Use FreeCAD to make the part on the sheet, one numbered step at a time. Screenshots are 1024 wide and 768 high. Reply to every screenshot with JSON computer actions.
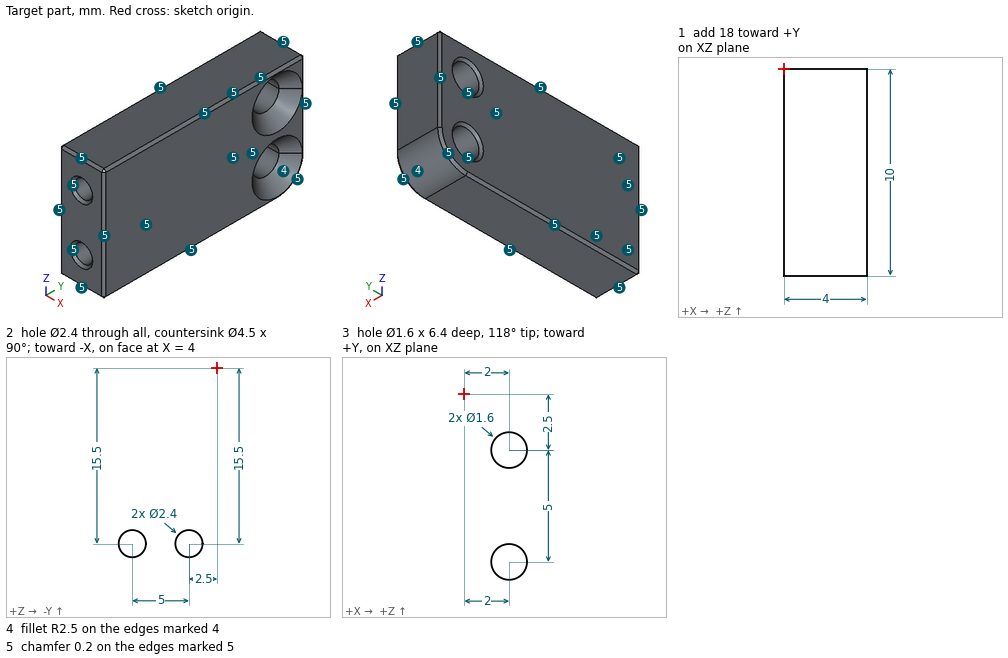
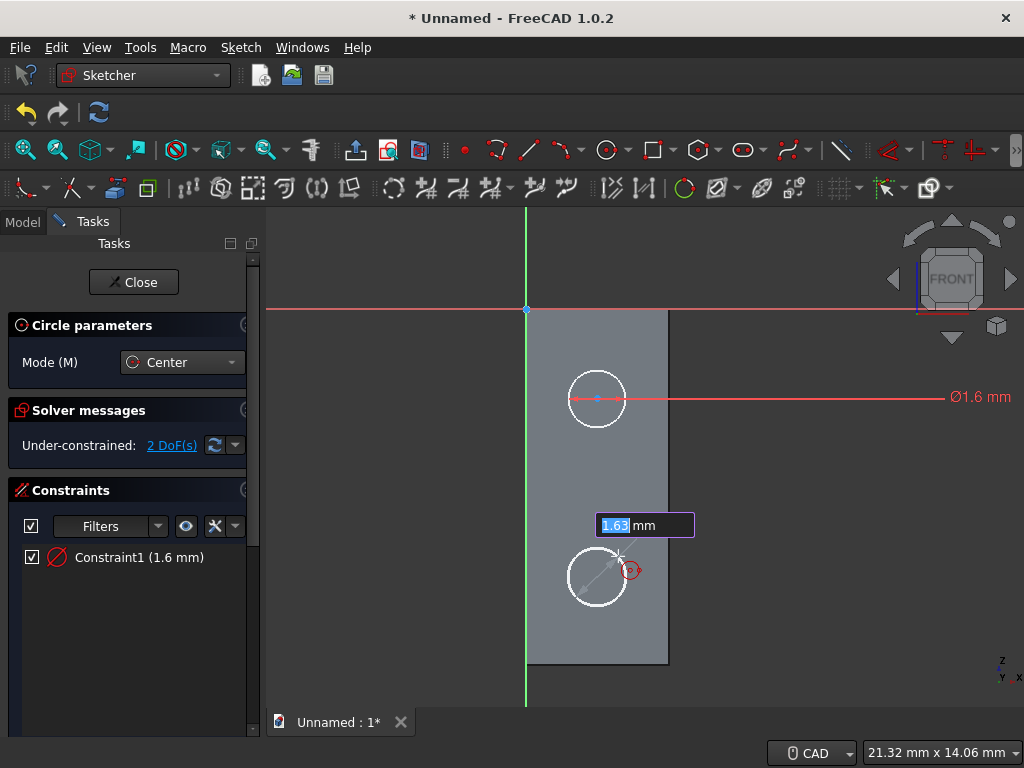
{"action": "type", "text": "1.6"}
{"action": "key", "text": "Return"}
{"action": "key", "text": "Escape"}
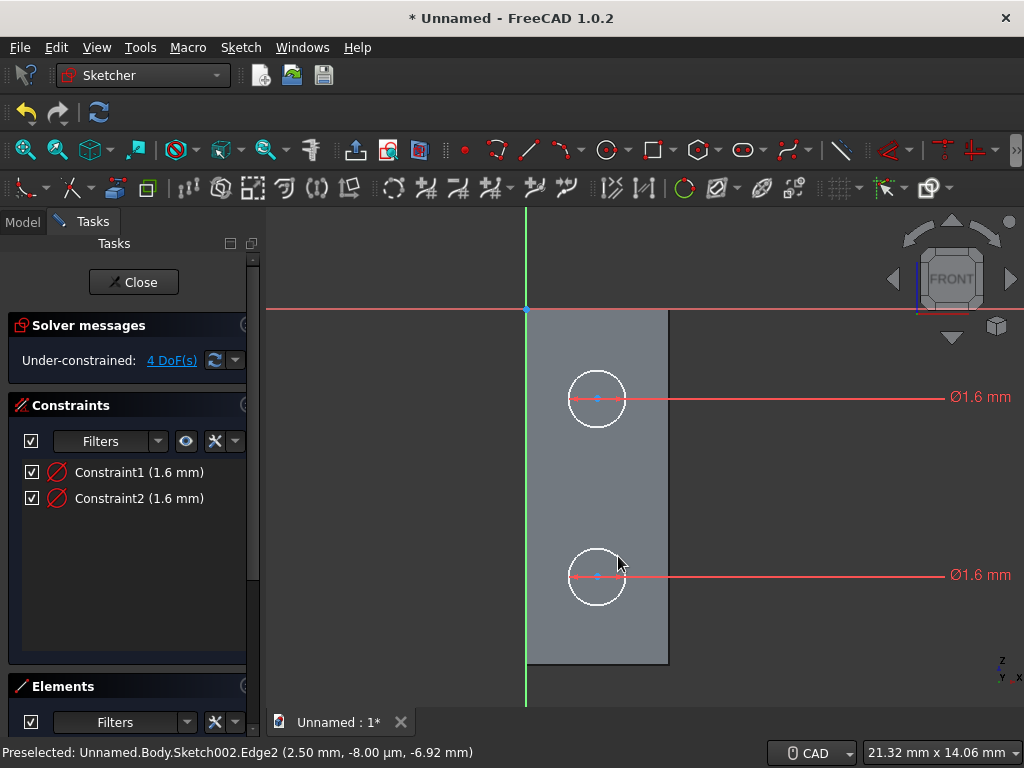
{"action": "left_click", "coordinate": [888, 150]}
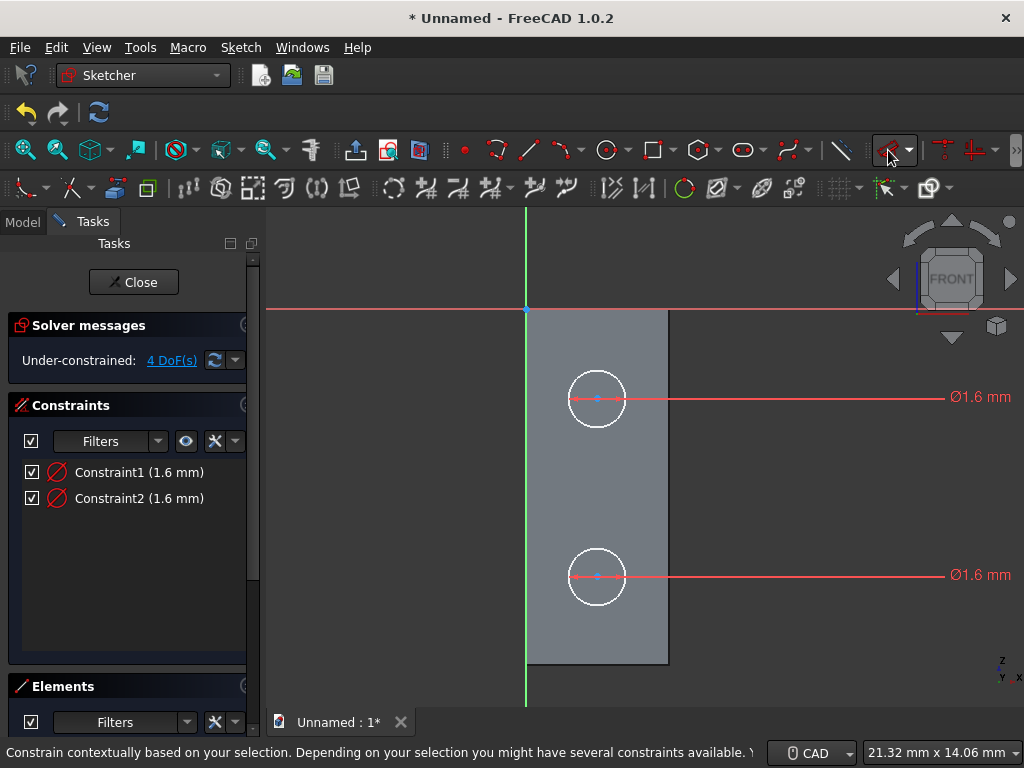
{"action": "left_click", "coordinate": [597, 399]}
{"action": "left_click", "coordinate": [562, 275]}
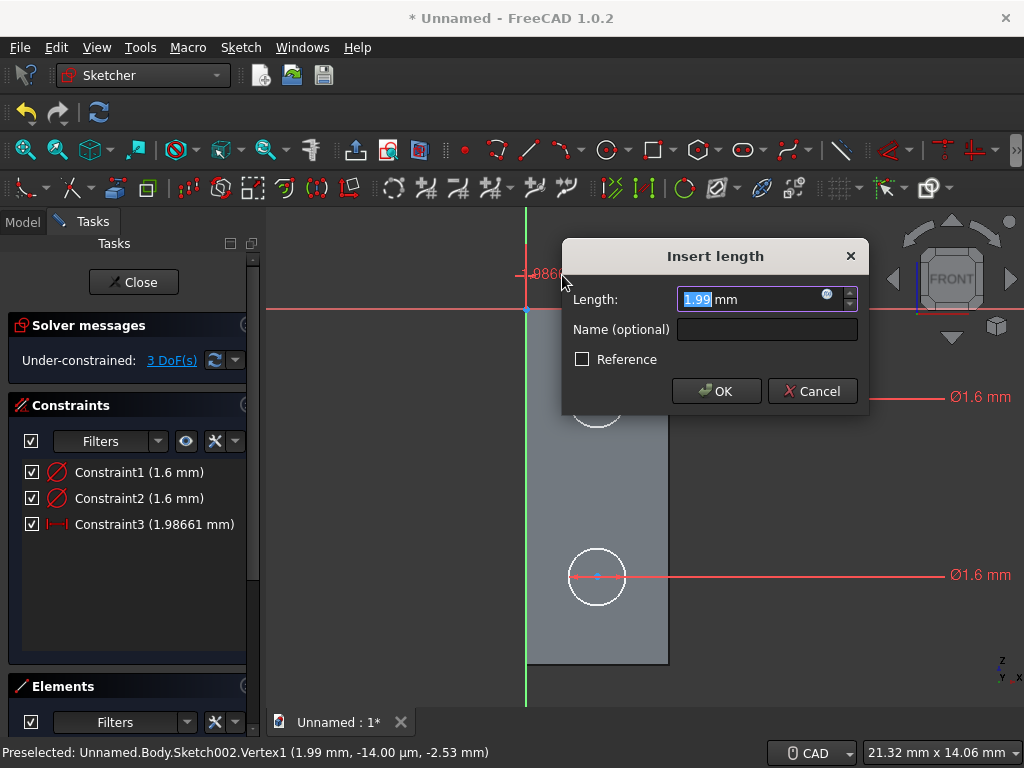
{"action": "type", "text": "2"}
{"action": "key", "text": "Return"}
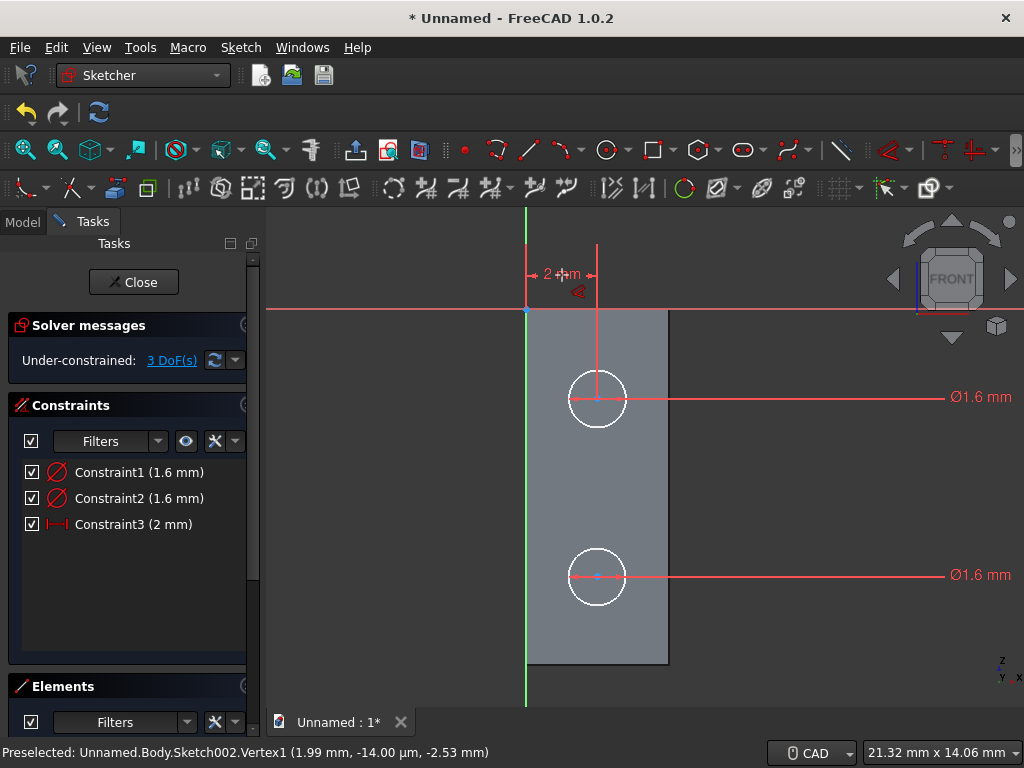
{"action": "left_click", "coordinate": [597, 577]}
{"action": "left_click", "coordinate": [562, 611]}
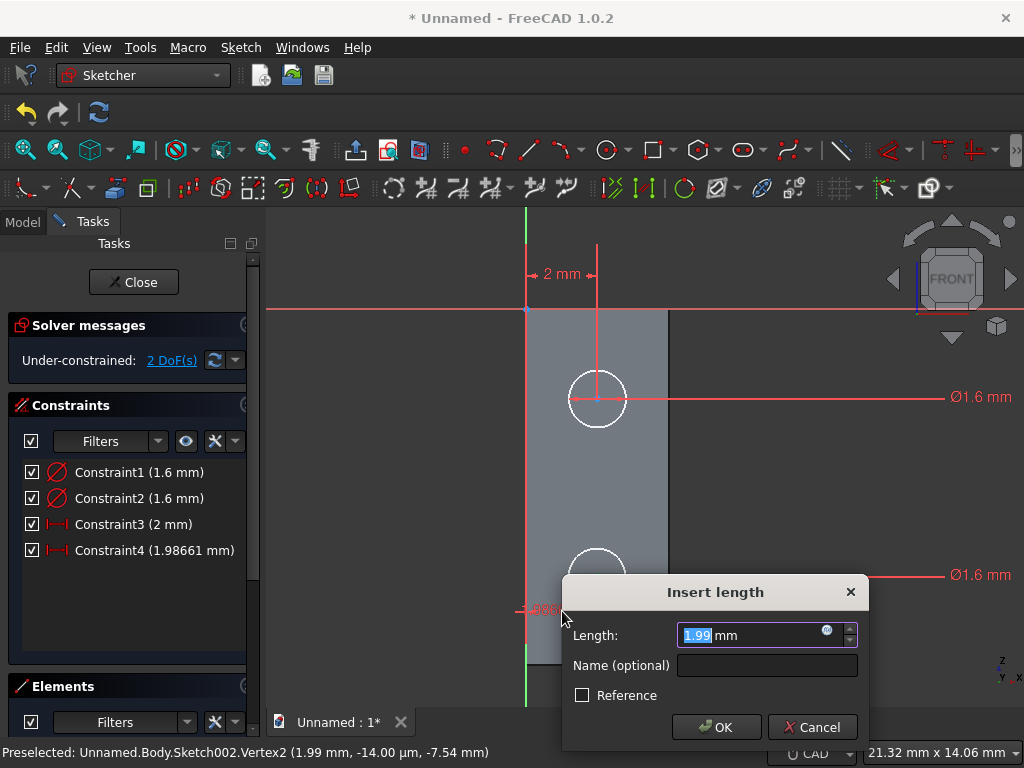
{"action": "type", "text": "2"}
{"action": "key", "text": "Return"}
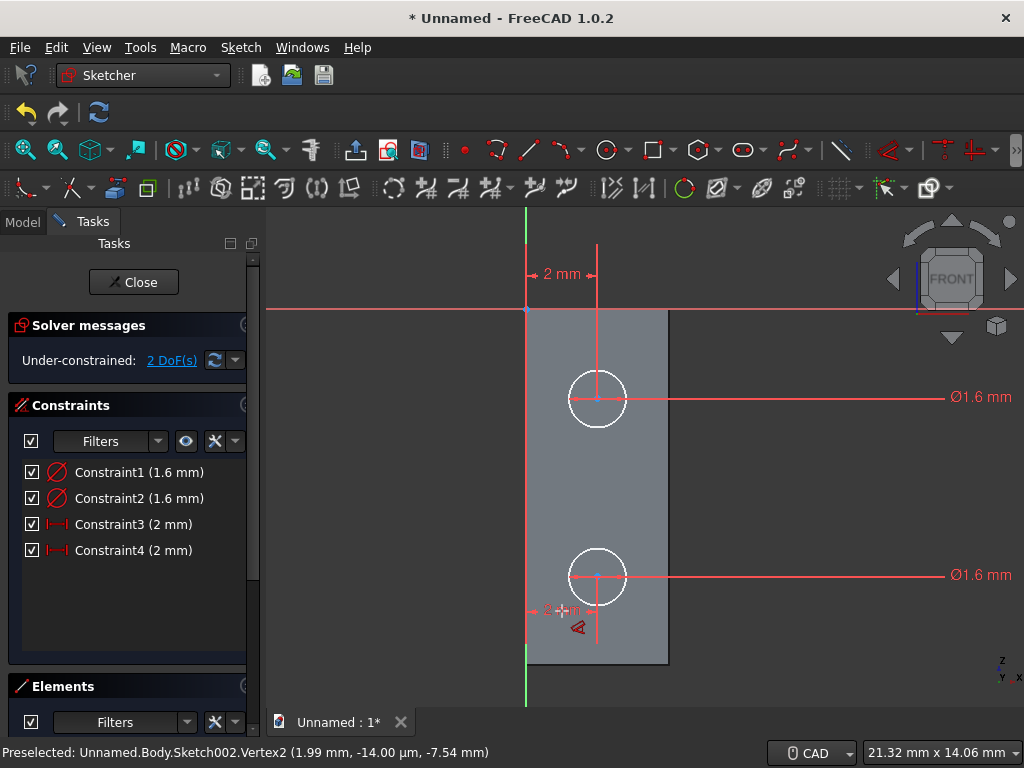
{"action": "left_click", "coordinate": [597, 399]}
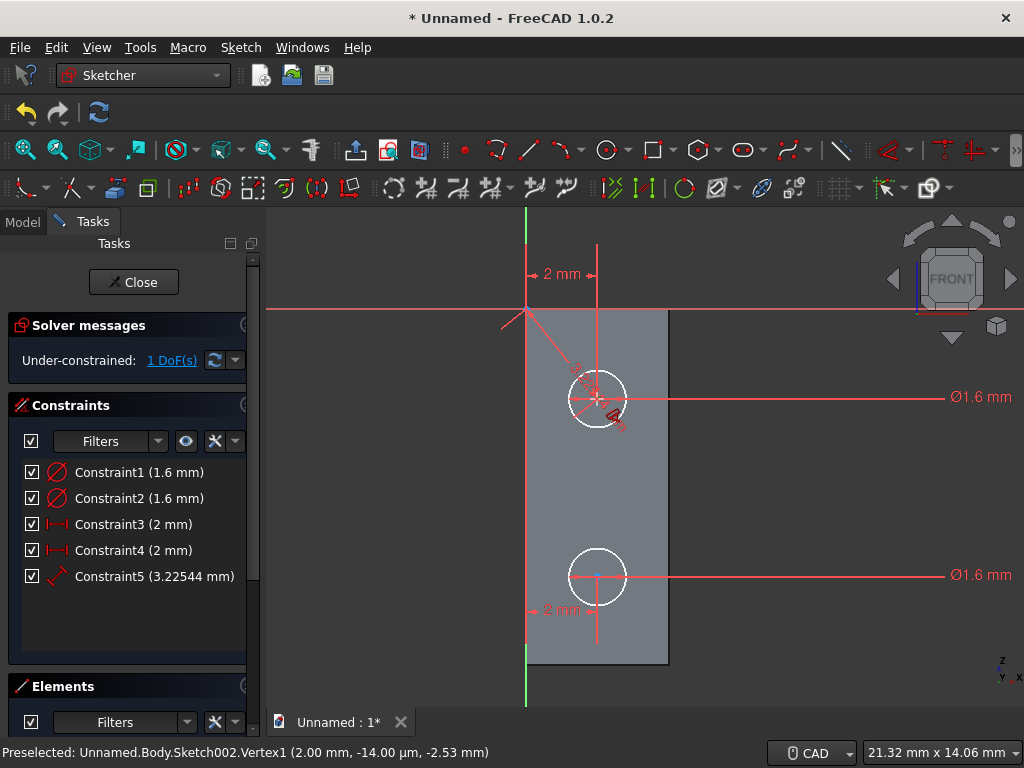
{"action": "left_click", "coordinate": [597, 577]}
{"action": "left_click", "coordinate": [631, 488]}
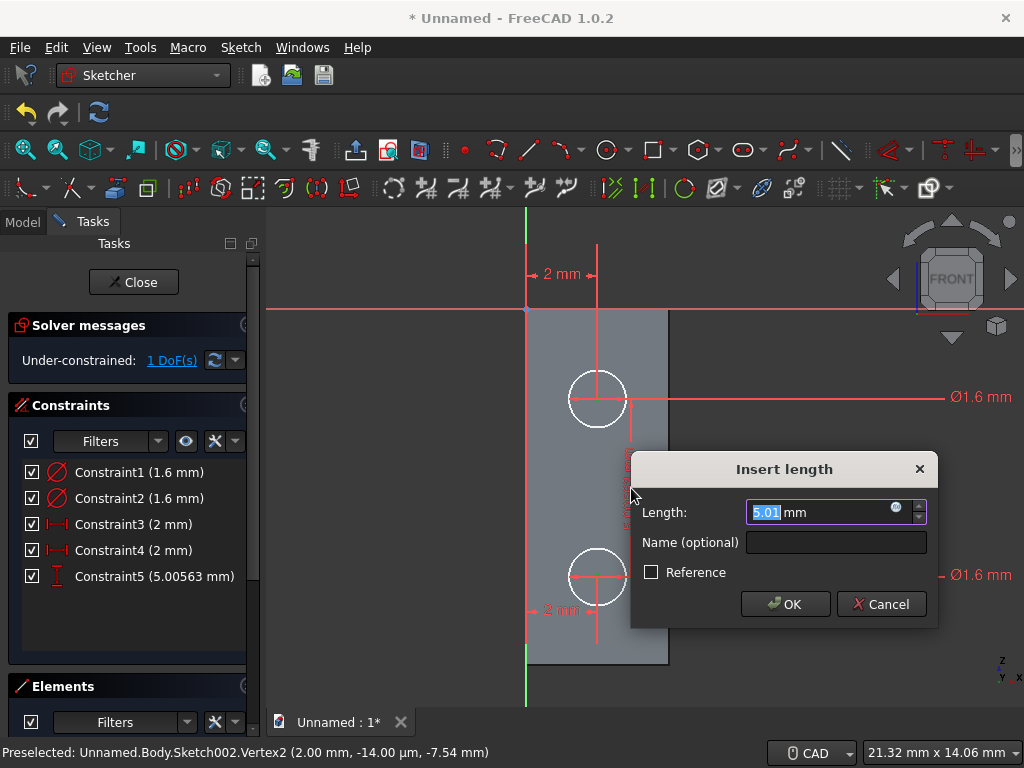
{"action": "type", "text": "5"}
{"action": "key", "text": "Return"}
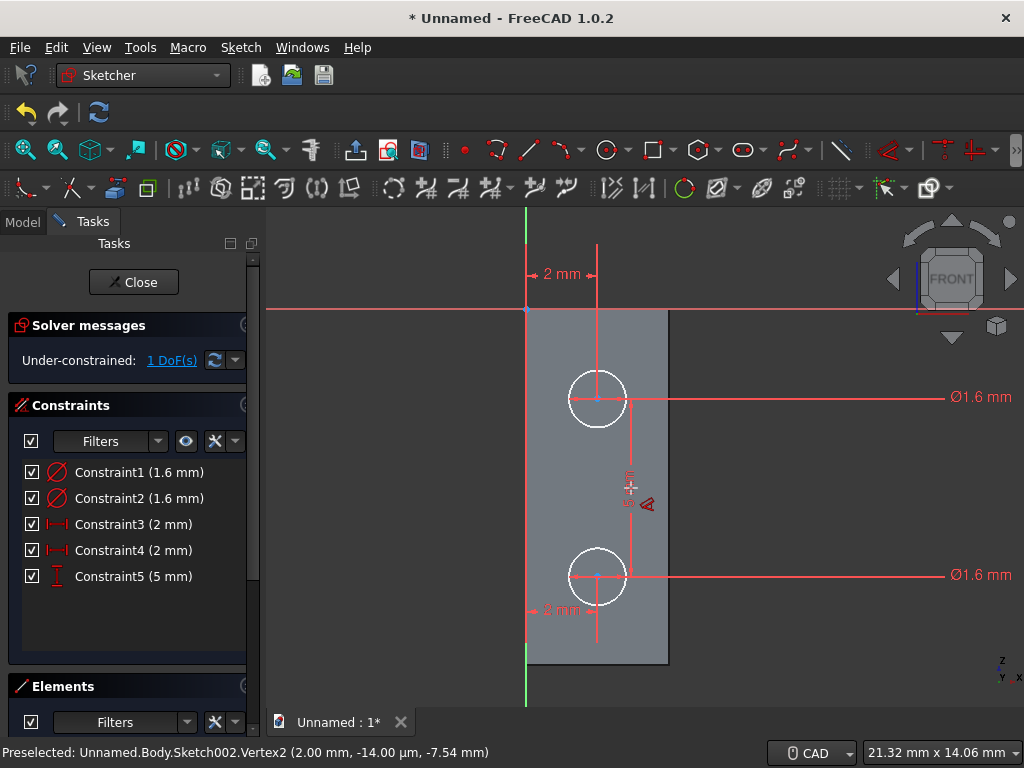
{"action": "left_click", "coordinate": [597, 399]}
{"action": "left_click", "coordinate": [492, 354]}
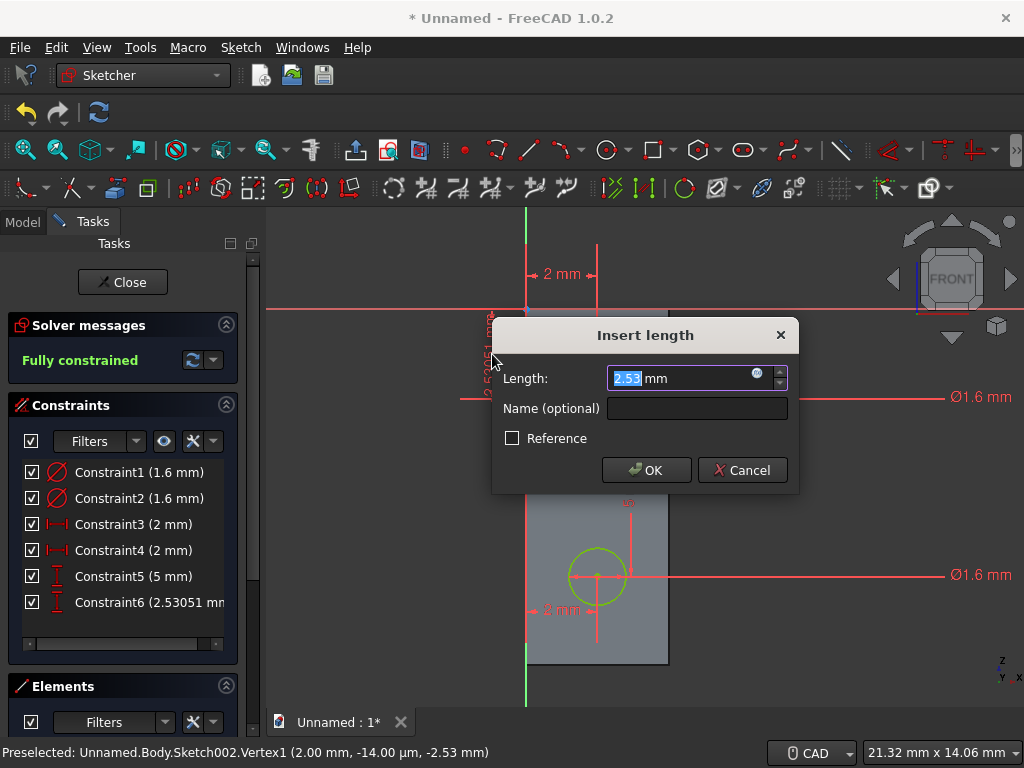
{"action": "type", "text": "2.5"}
{"action": "key", "text": "Return"}
{"action": "key", "text": "Escape"}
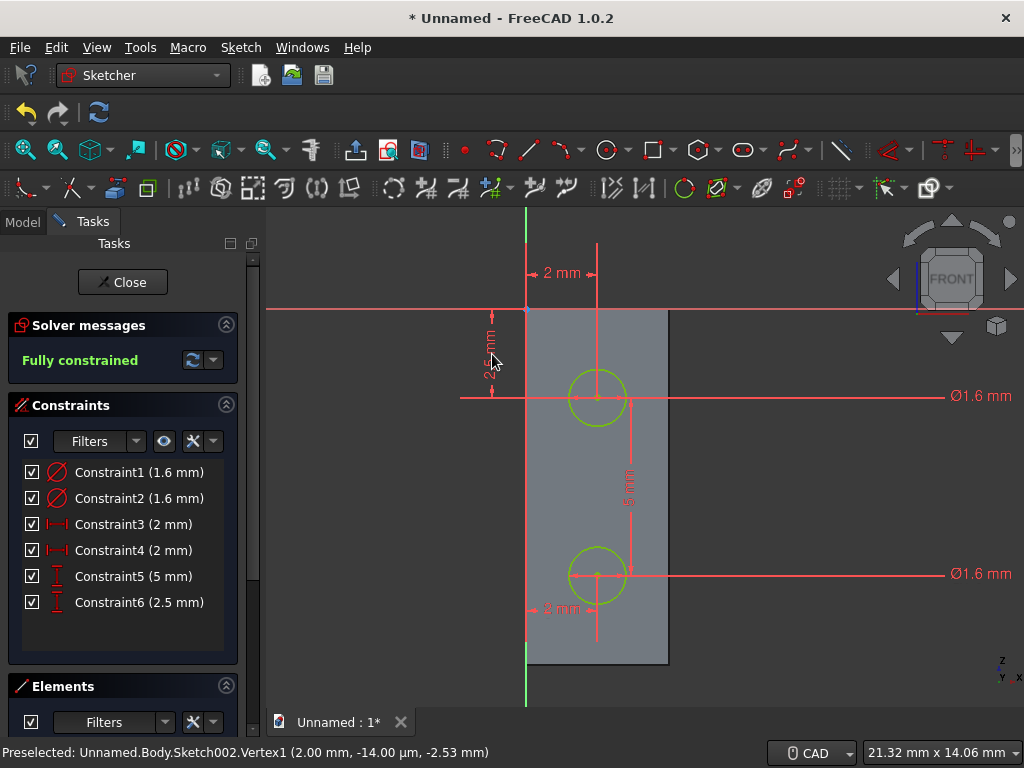
{"action": "left_click", "coordinate": [123, 282]}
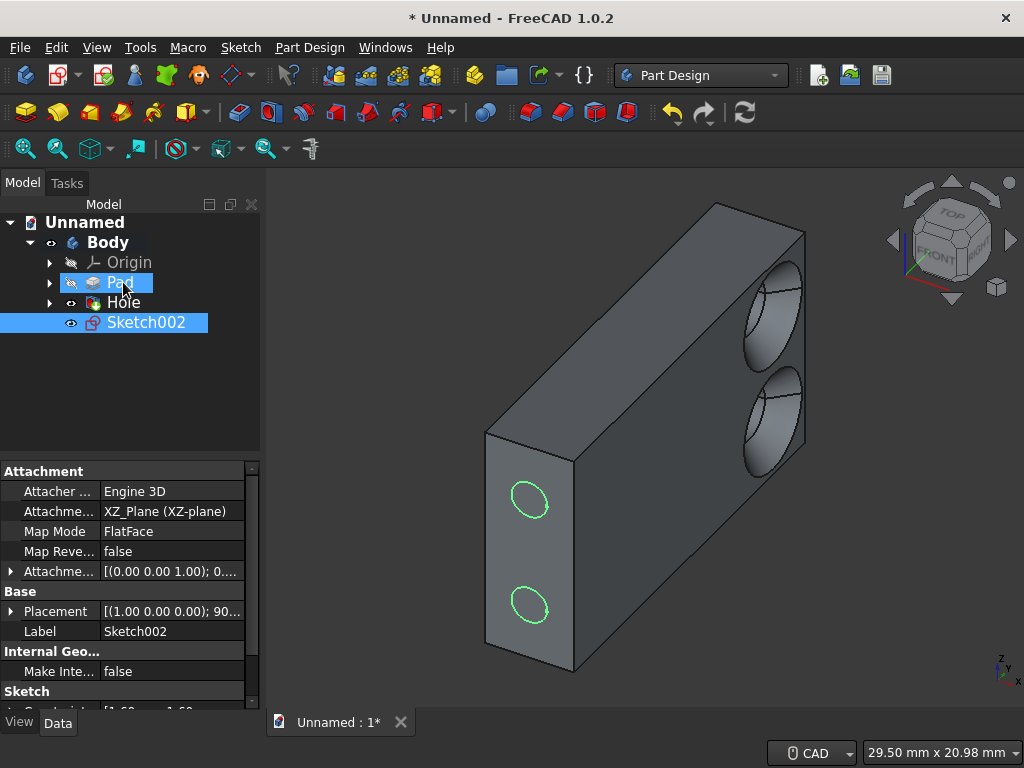
{"action": "left_click", "coordinate": [272, 112]}